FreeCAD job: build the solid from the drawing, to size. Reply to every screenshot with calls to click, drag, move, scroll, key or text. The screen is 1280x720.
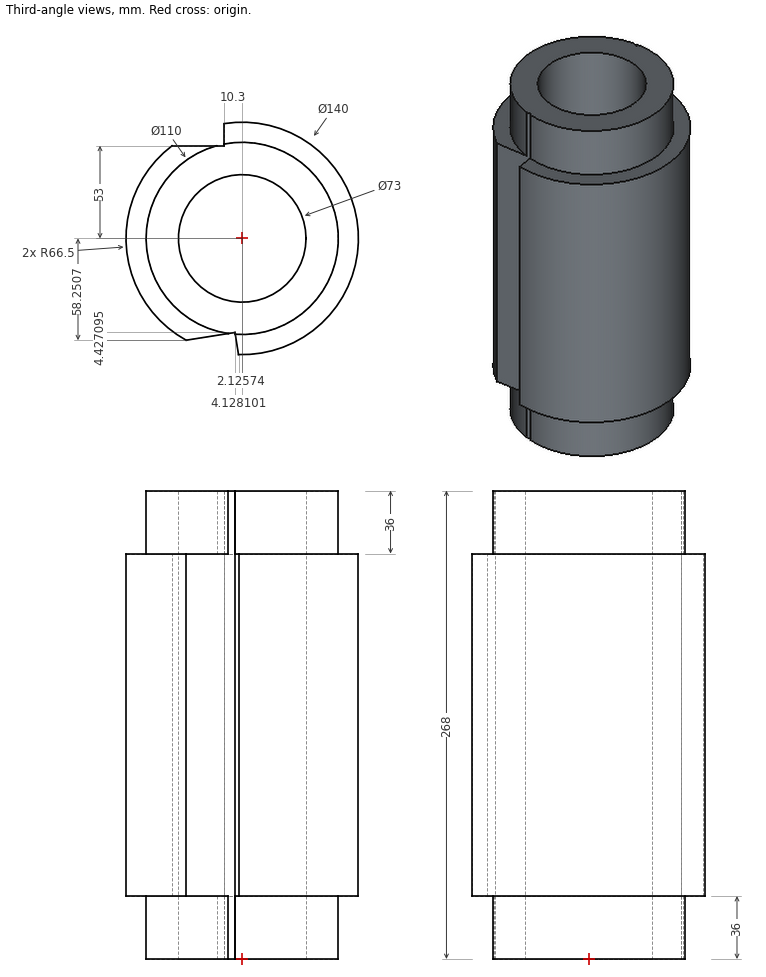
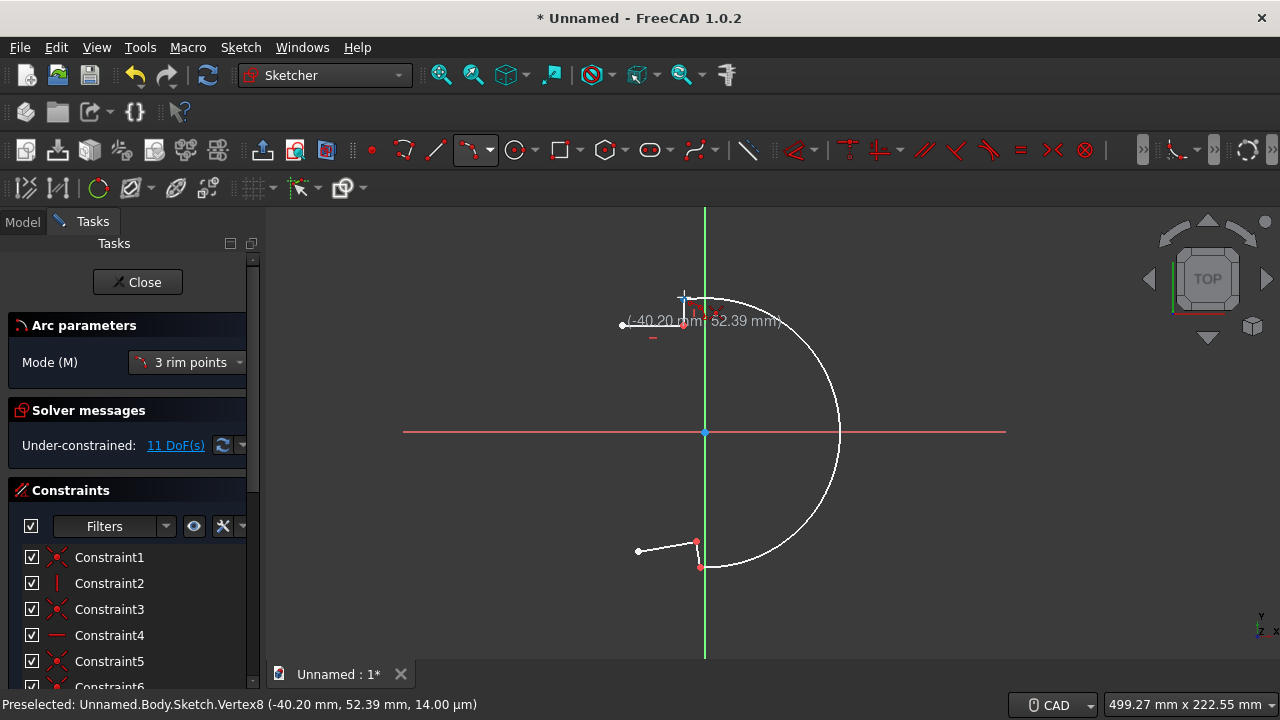
click(639, 552)
click(571, 415)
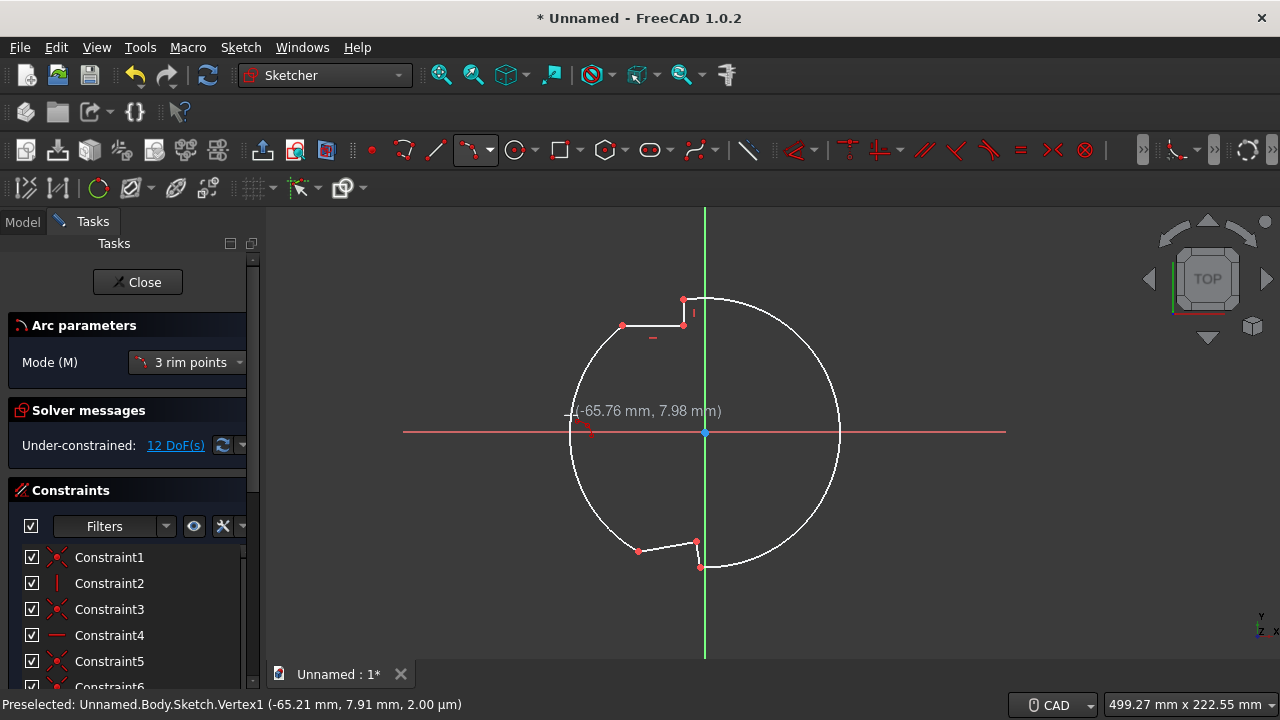
click(516, 150)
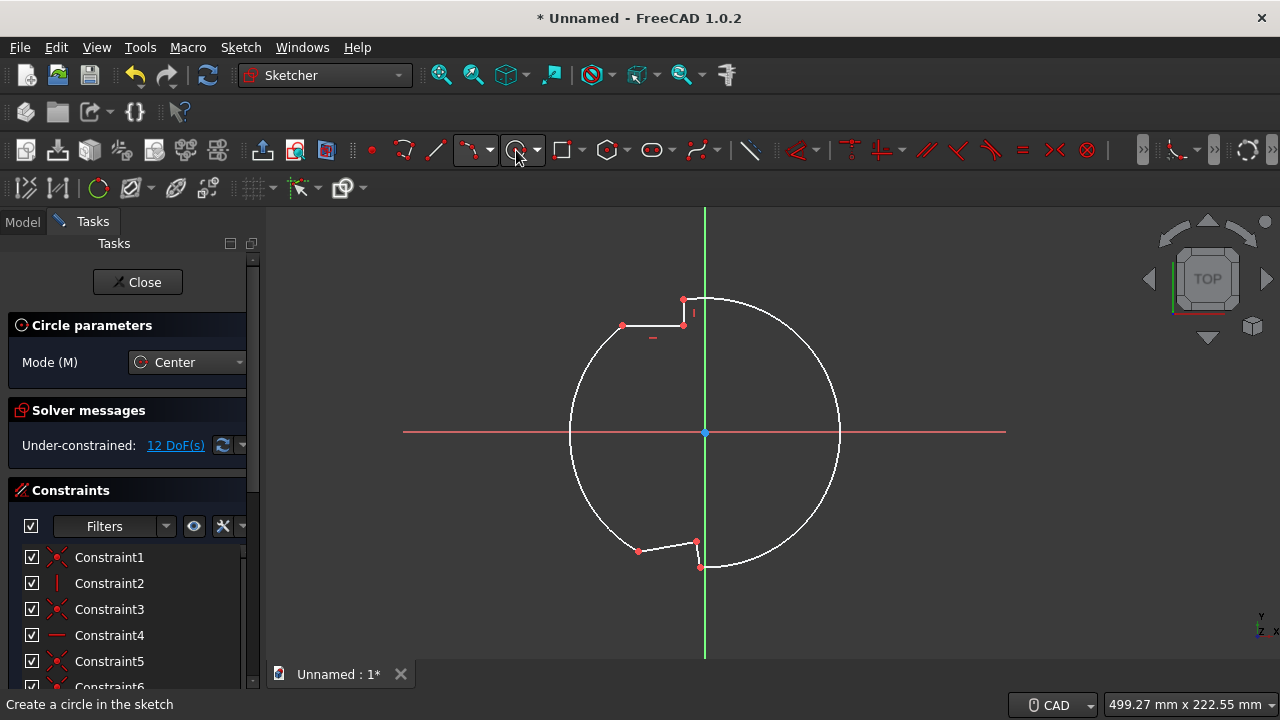
click(705, 432)
click(757, 380)
key(Escape)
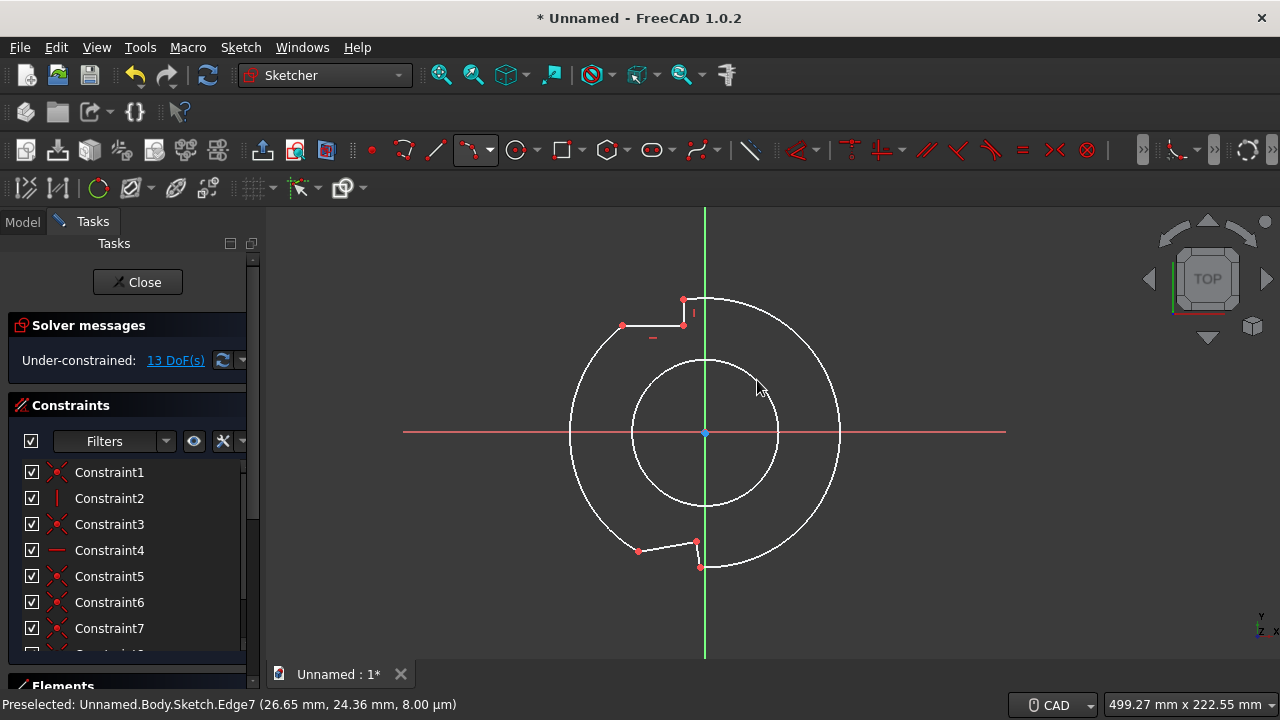
click(757, 381)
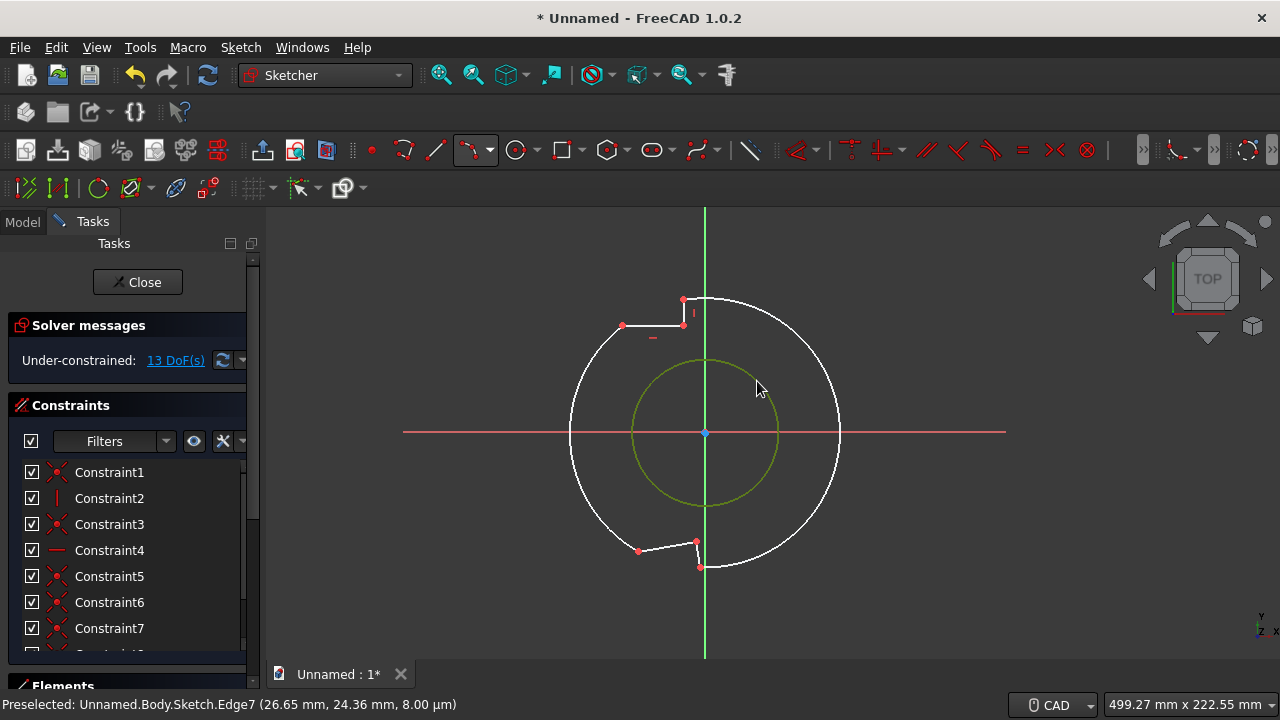
click(577, 390)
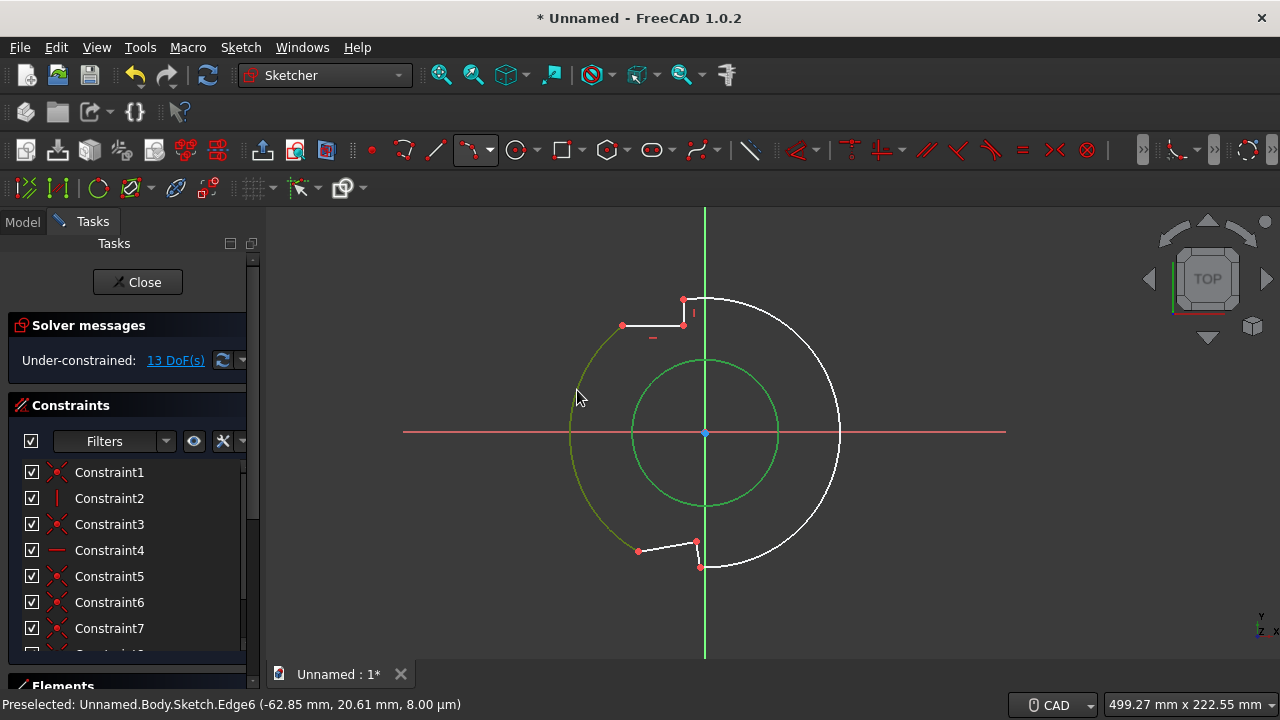
click(850, 150)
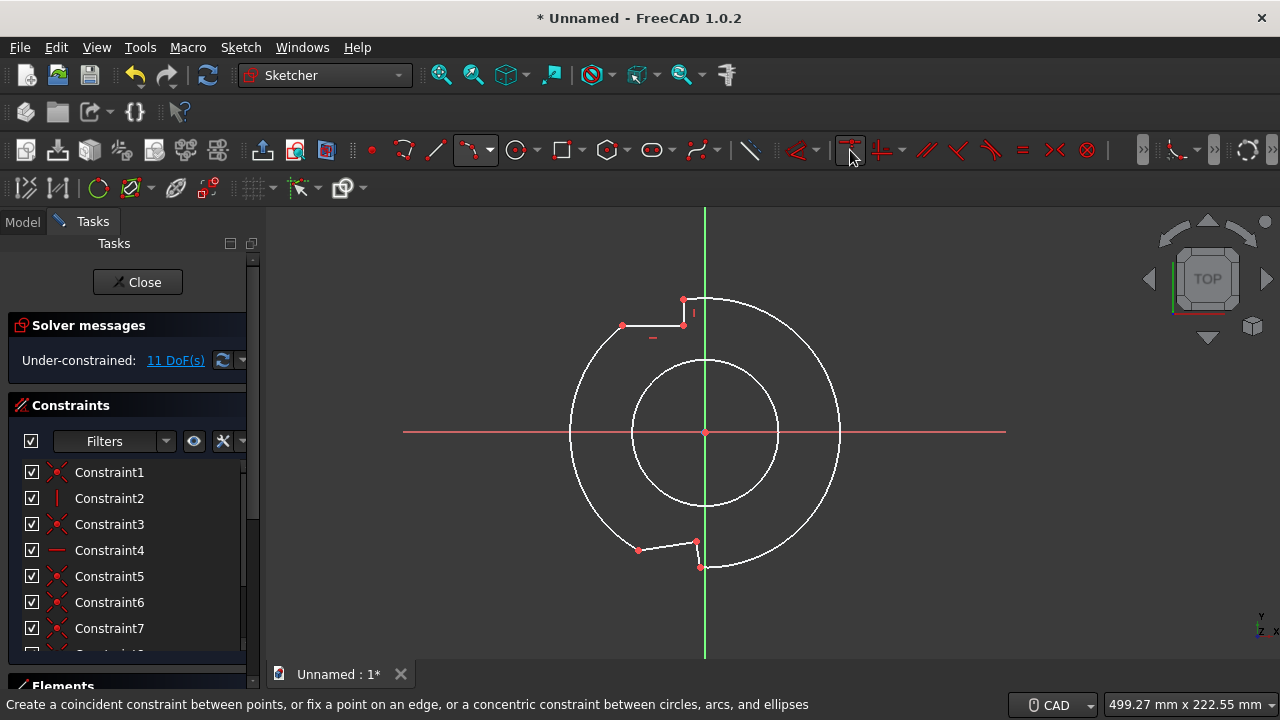
drag(695, 422, 715, 443)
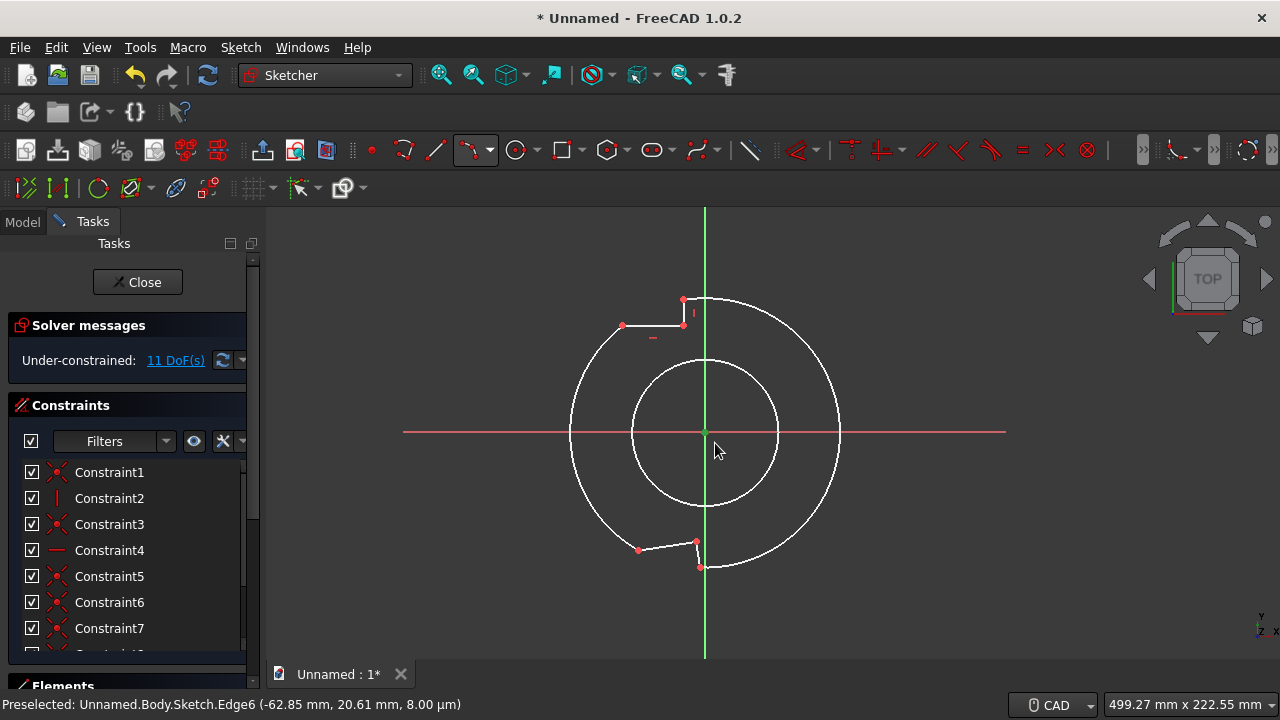
key(c)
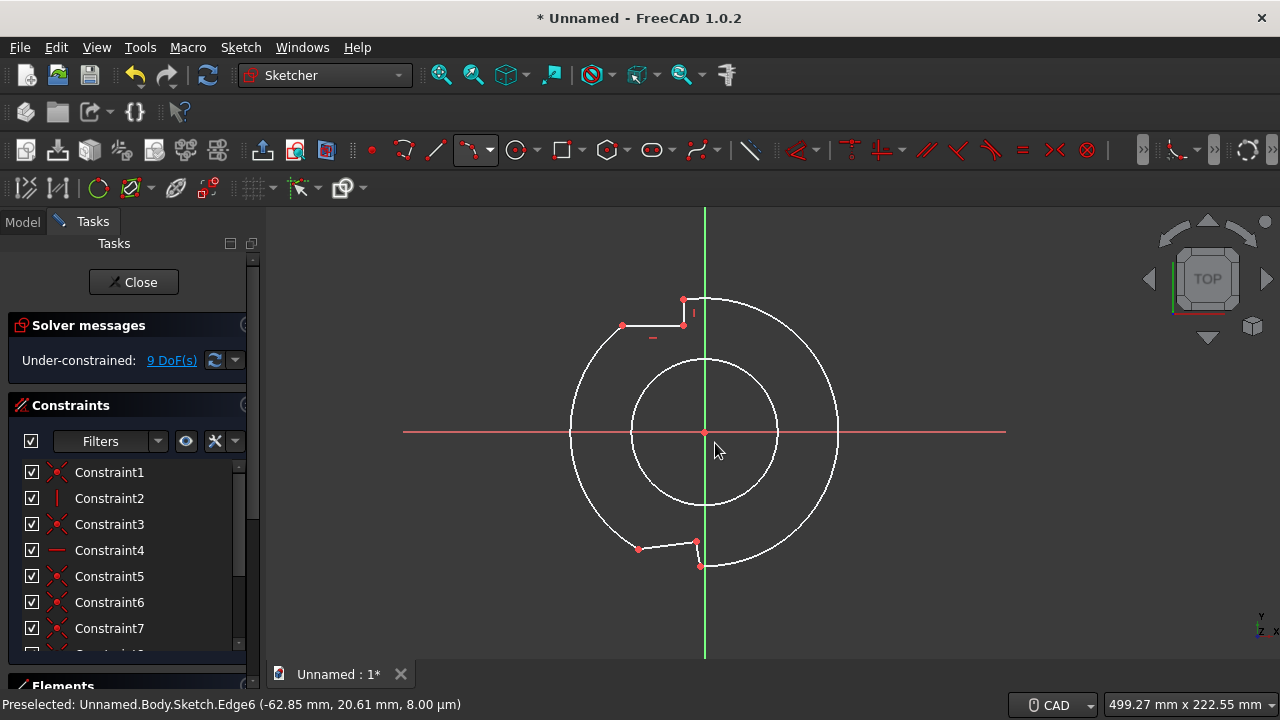
click(815, 508)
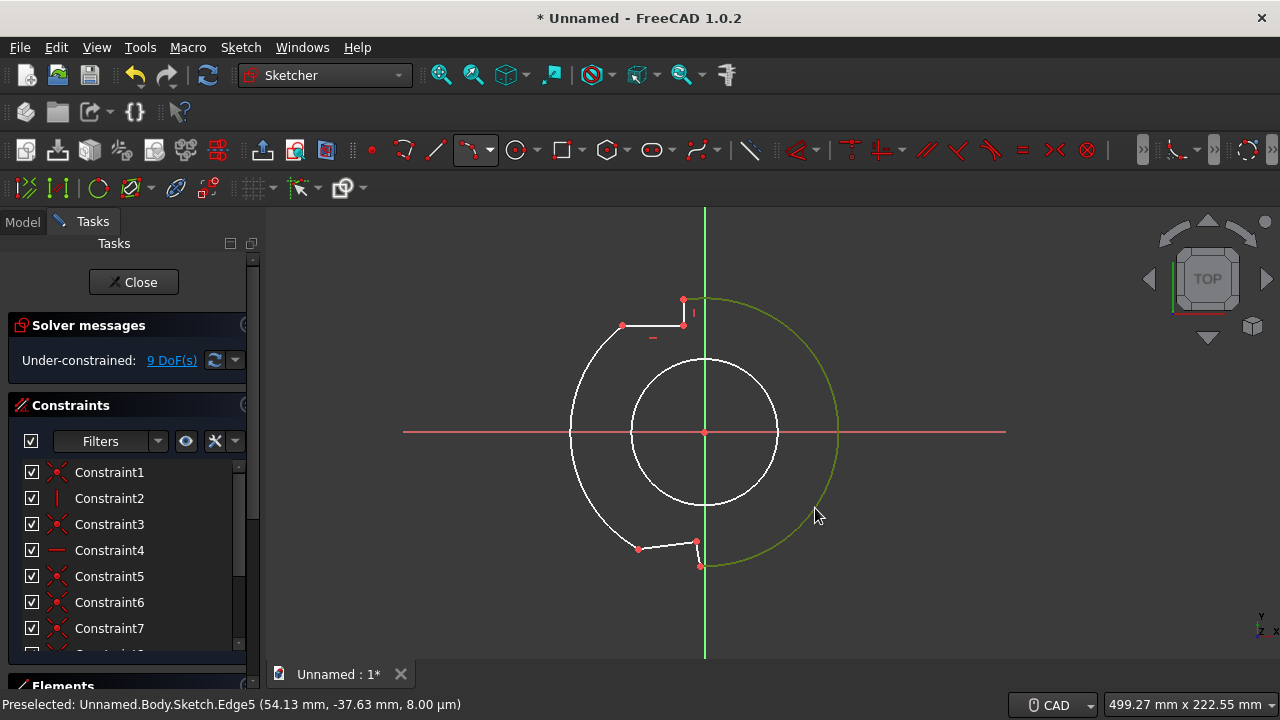
click(577, 390)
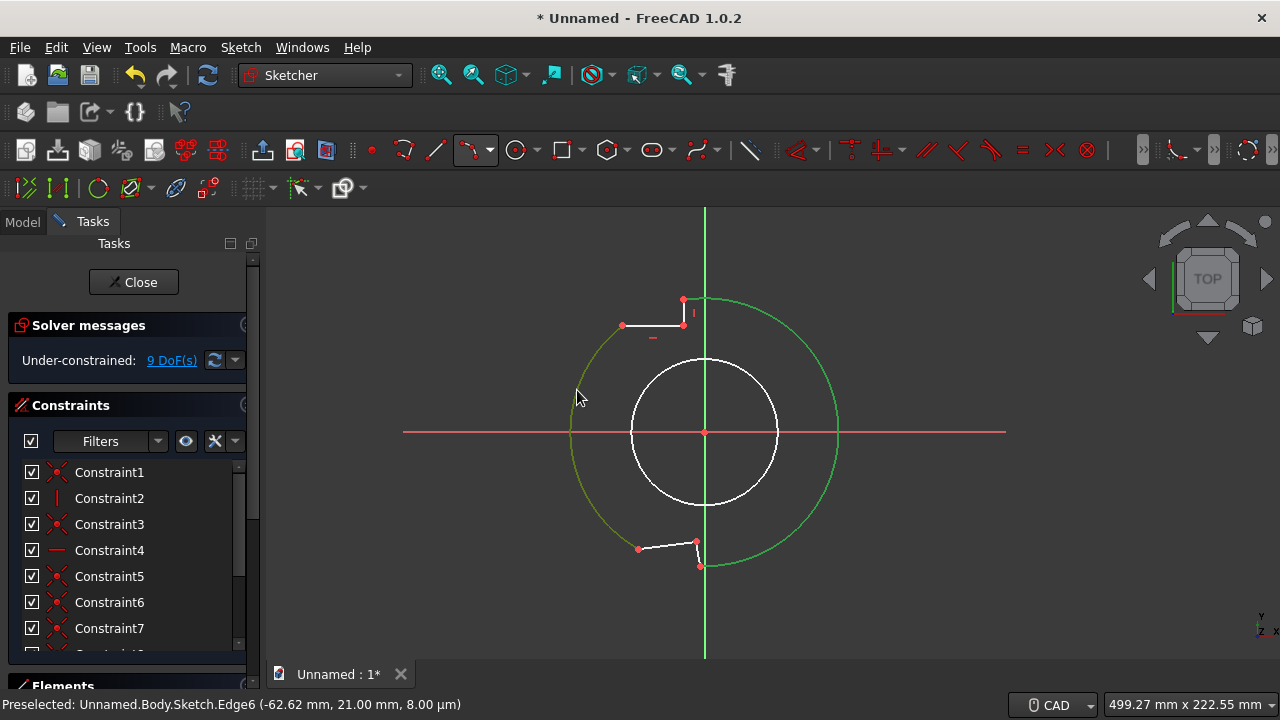
click(1024, 150)